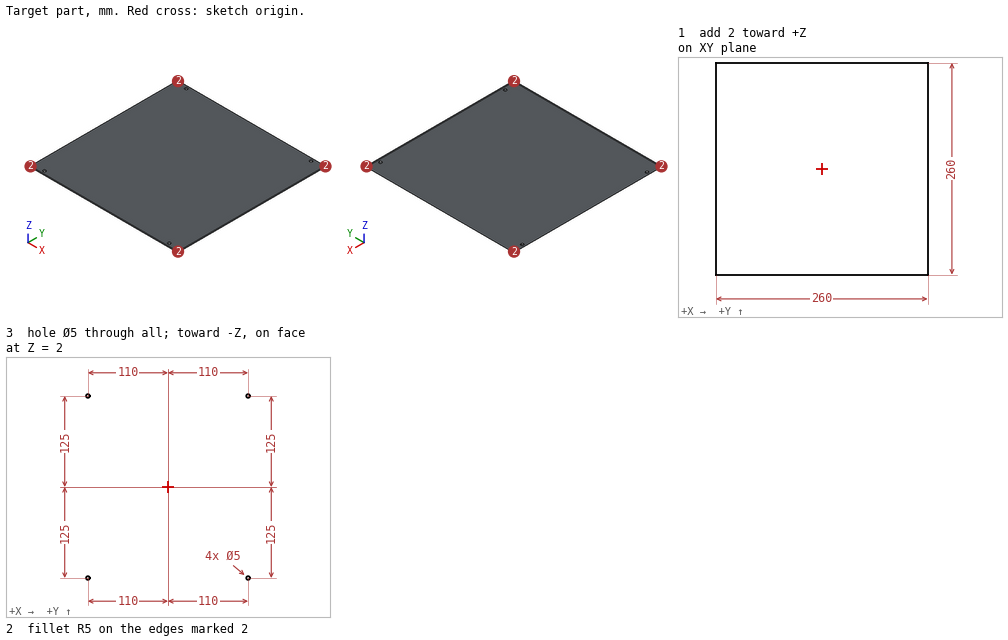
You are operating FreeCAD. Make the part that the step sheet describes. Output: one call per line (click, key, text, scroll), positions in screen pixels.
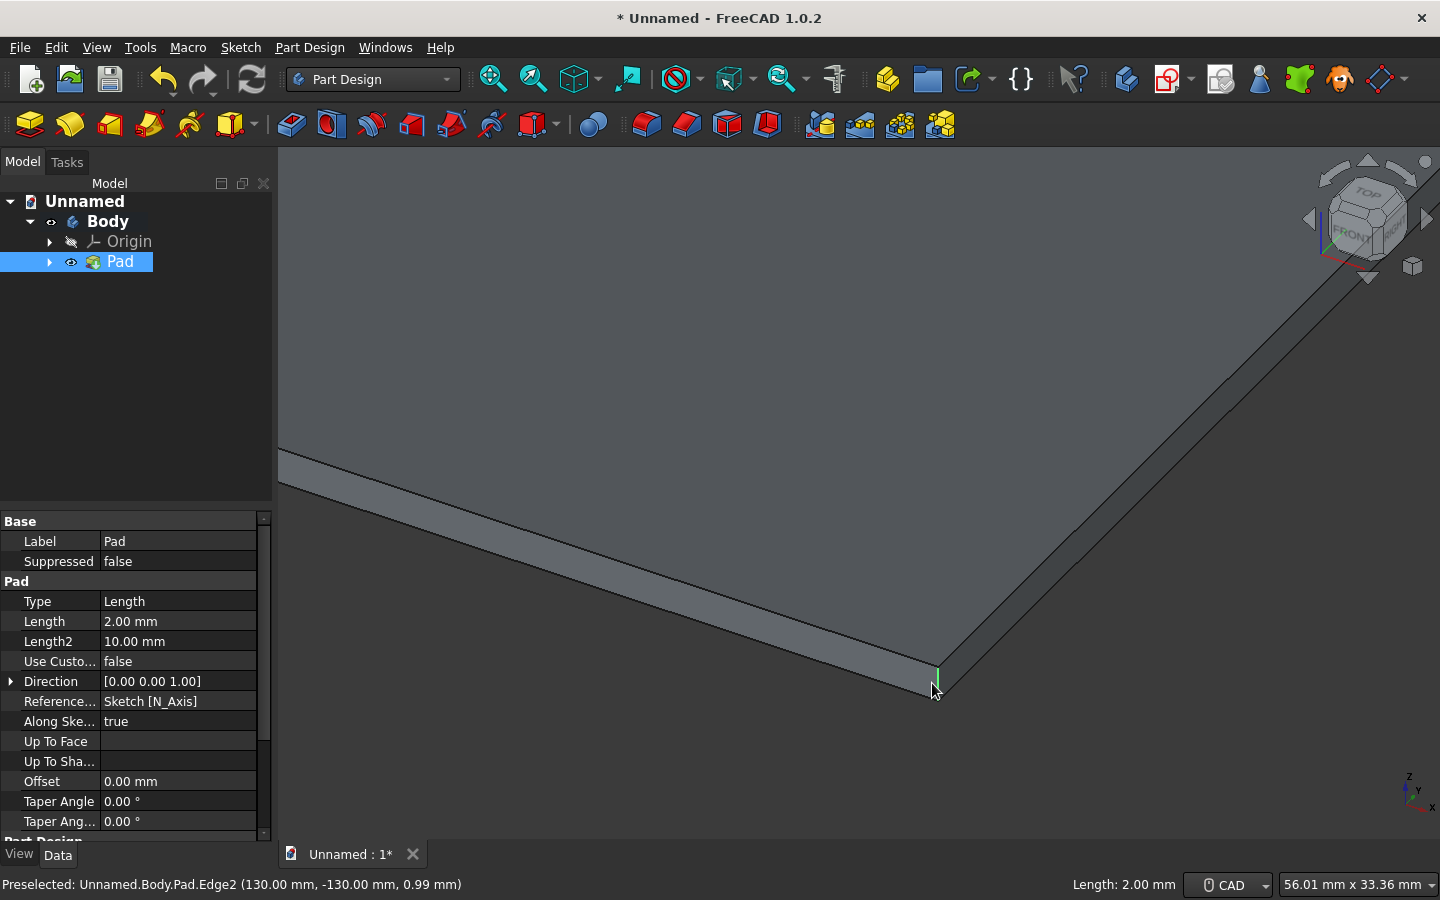
key(v)
key(f)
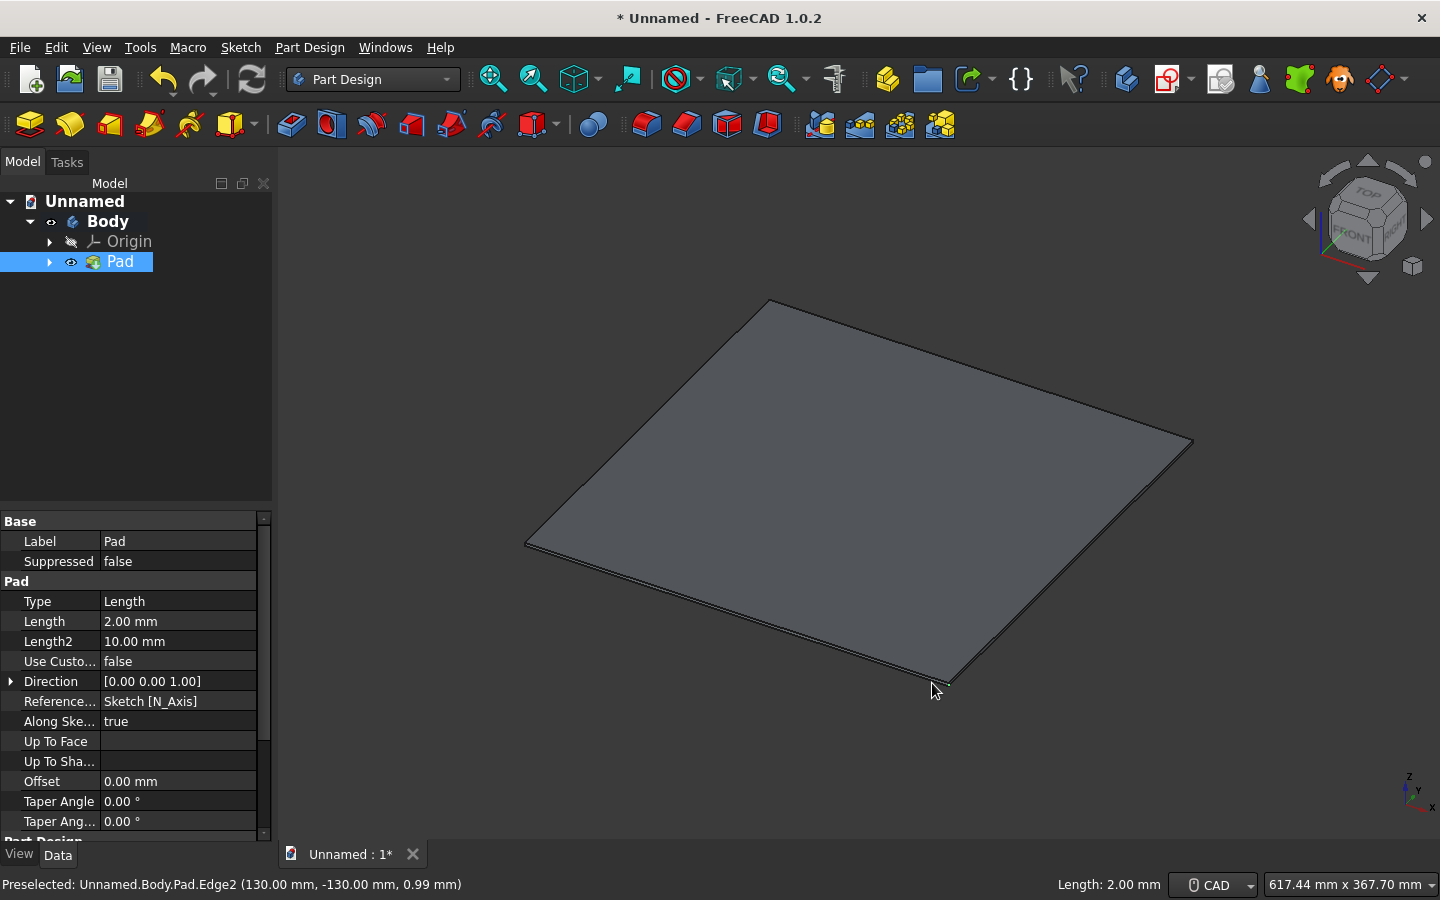
key(0)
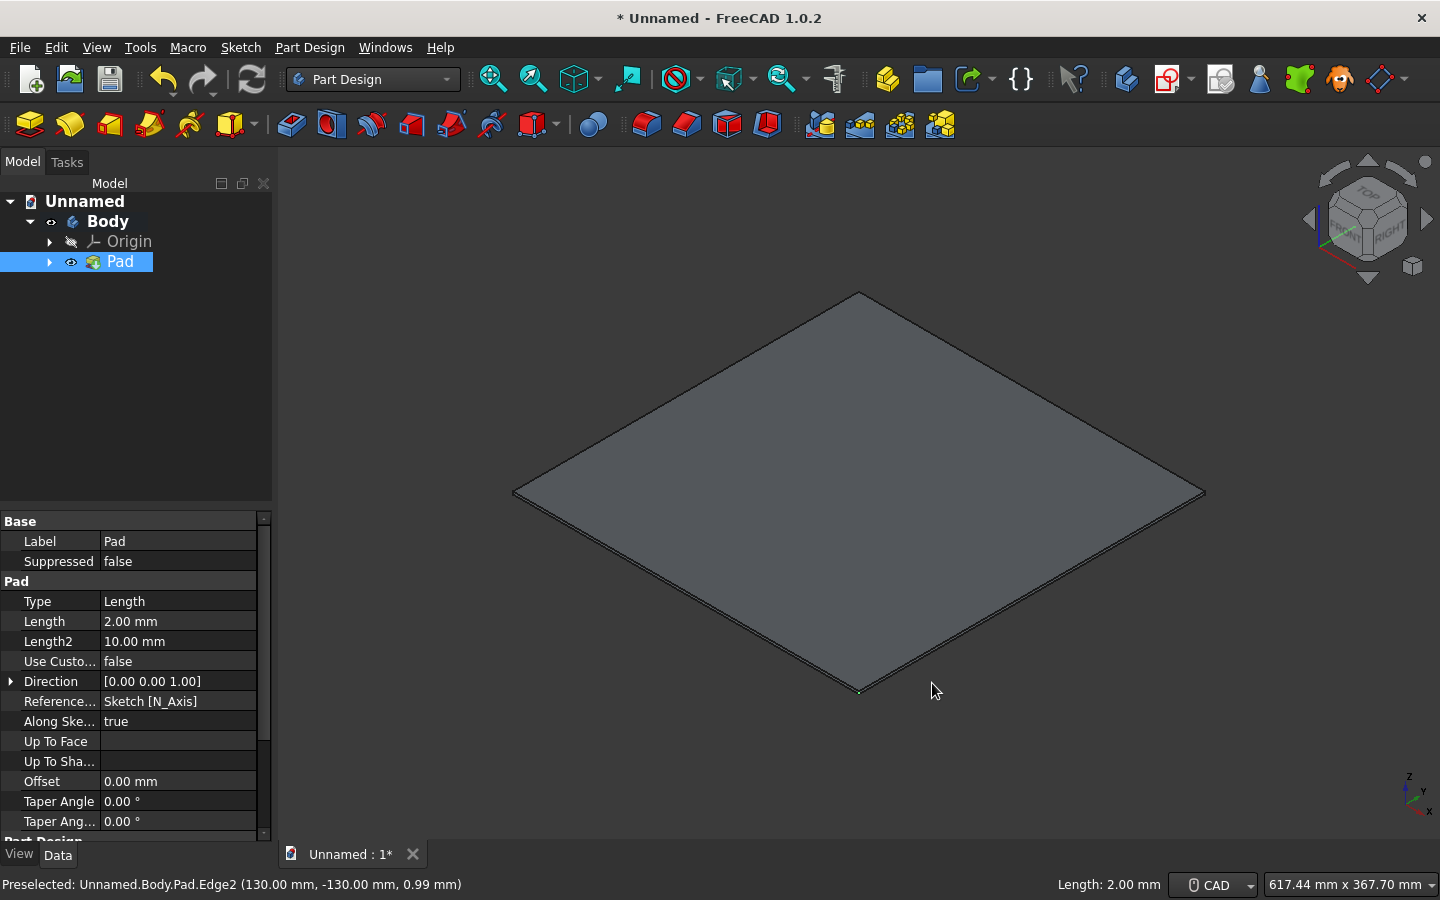
scroll(513, 492, up, 12)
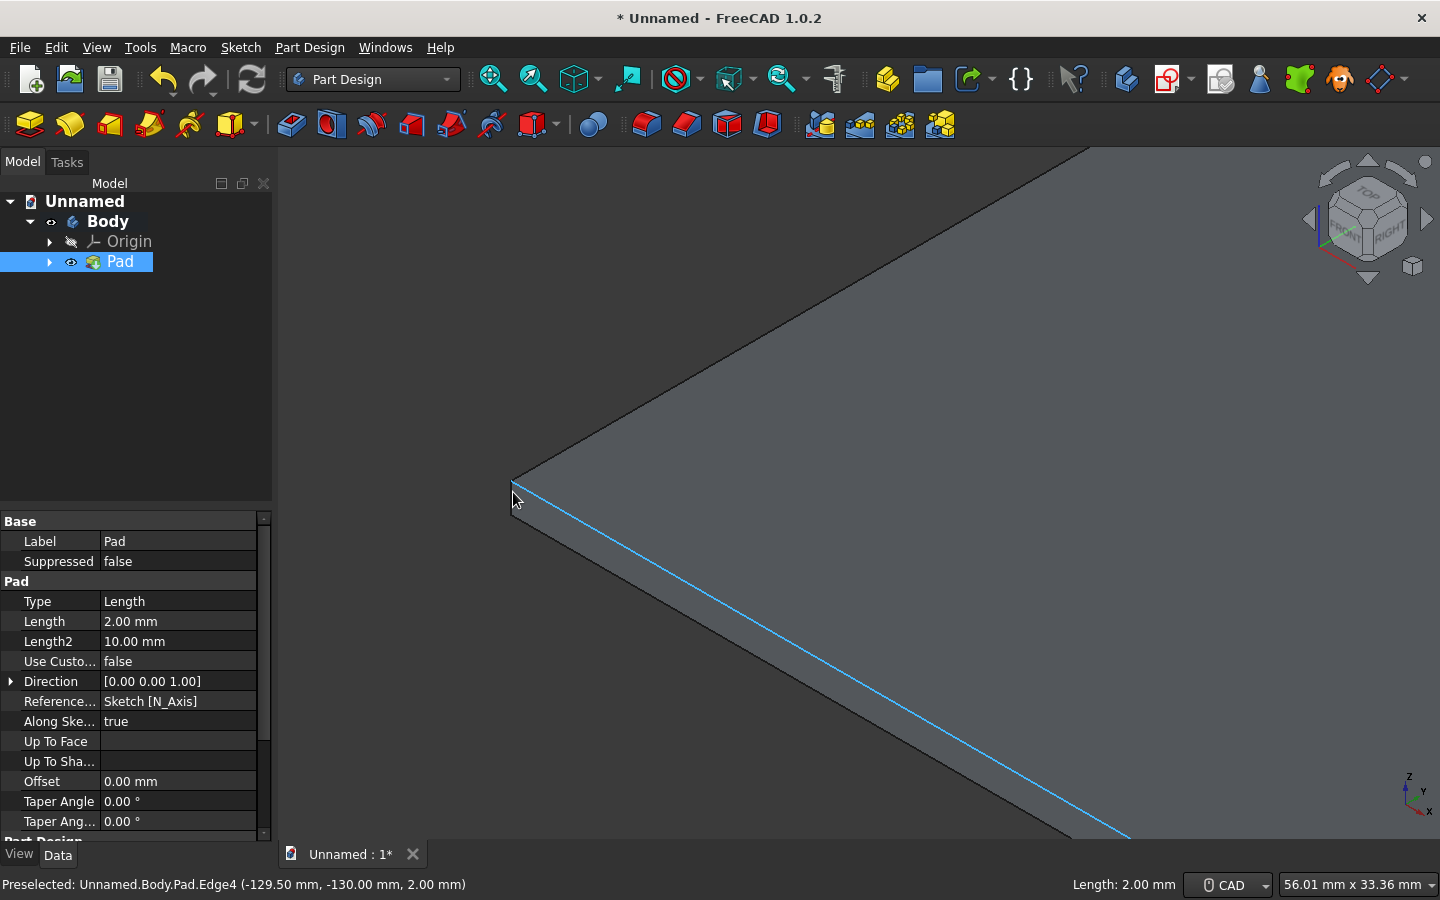
key(v)
key(f)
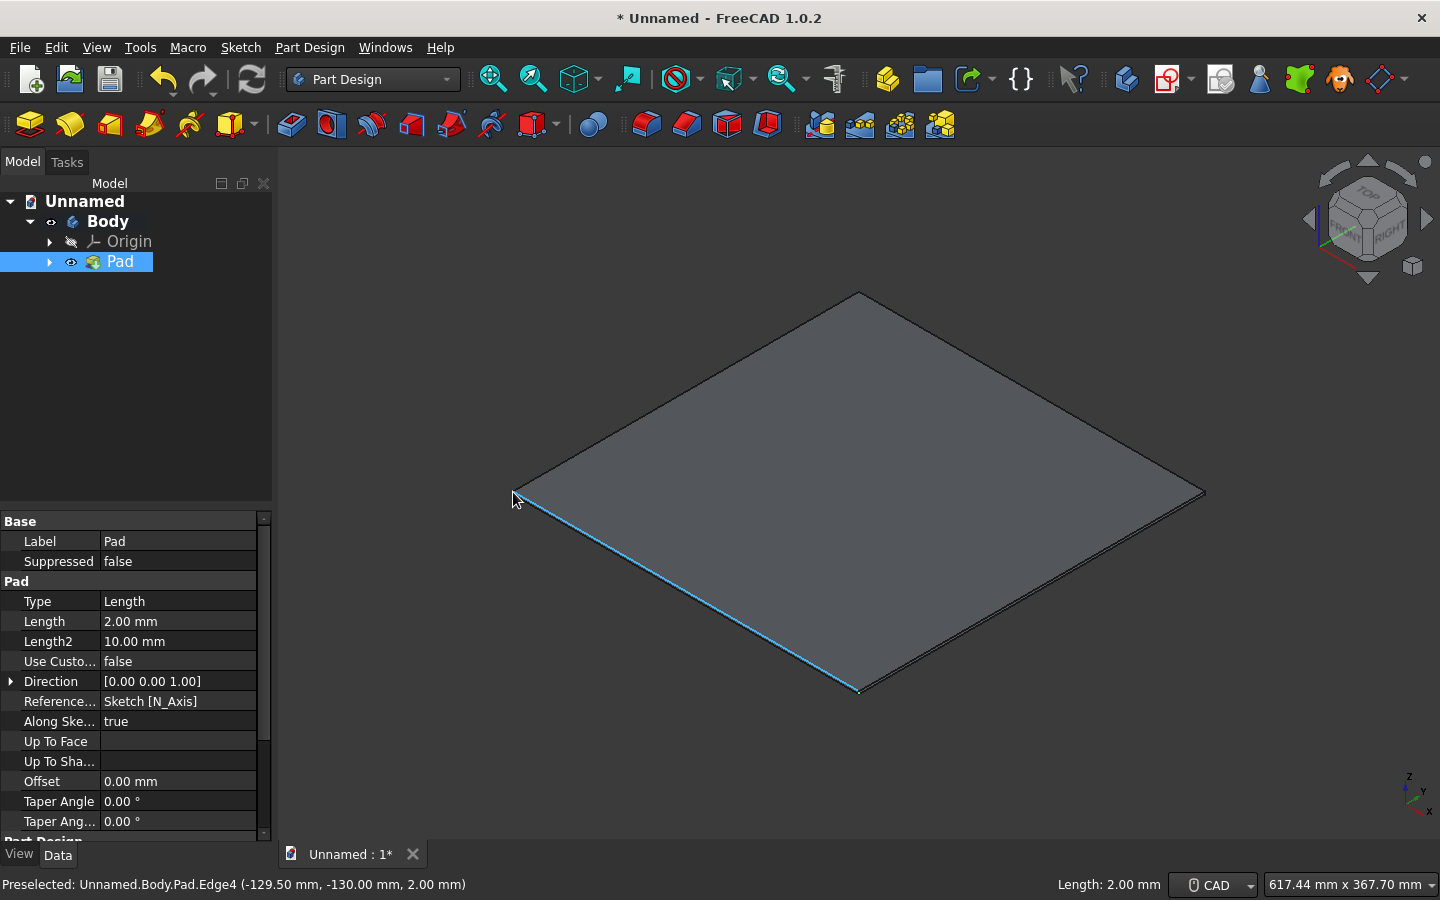
key(2)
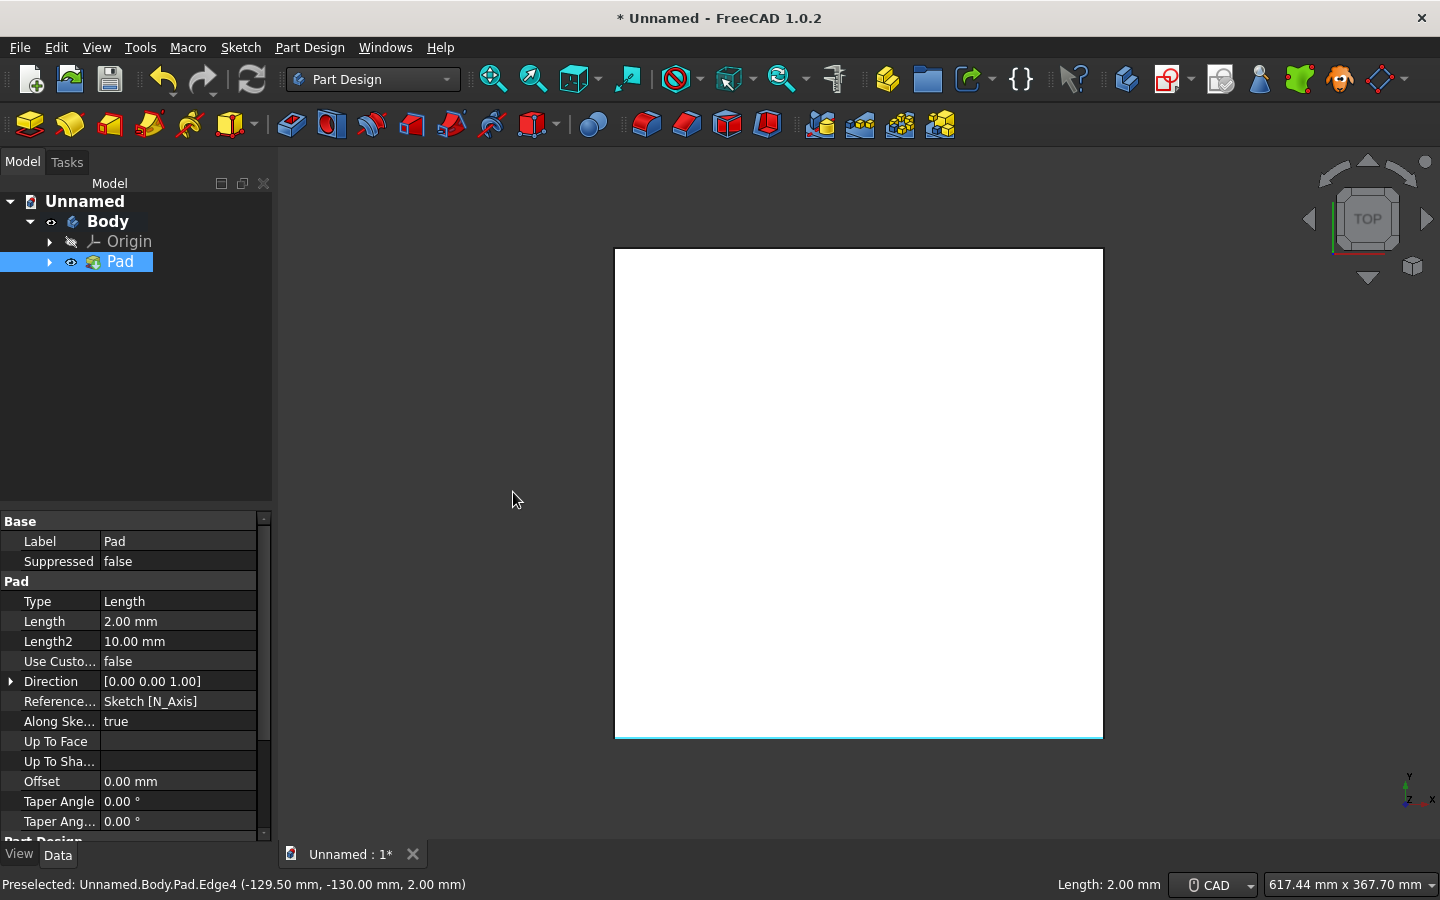
scroll(614, 737, up, 12)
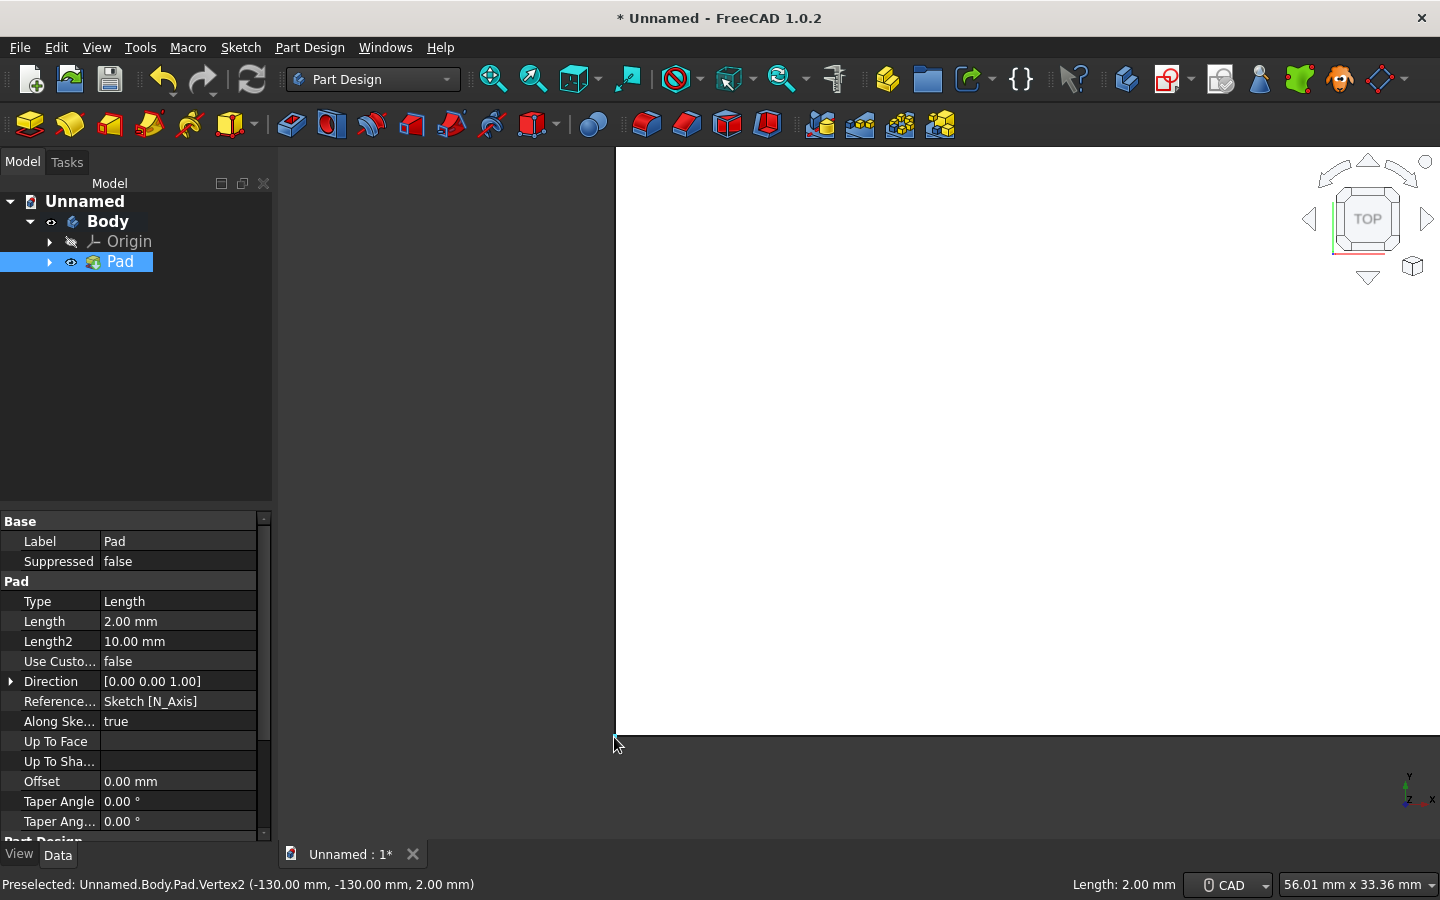
click(494, 80)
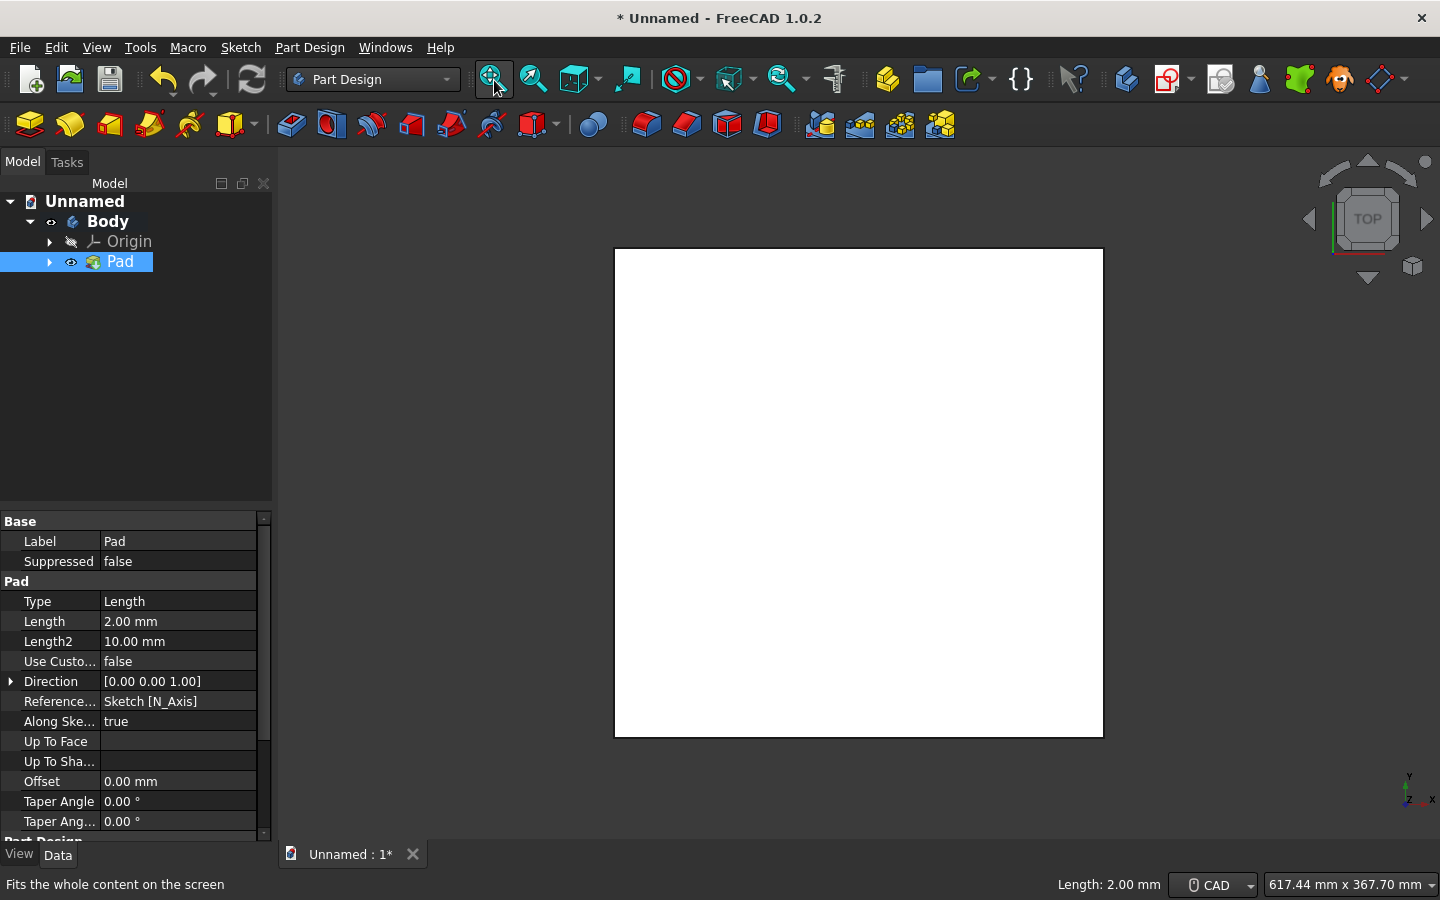
key(1)